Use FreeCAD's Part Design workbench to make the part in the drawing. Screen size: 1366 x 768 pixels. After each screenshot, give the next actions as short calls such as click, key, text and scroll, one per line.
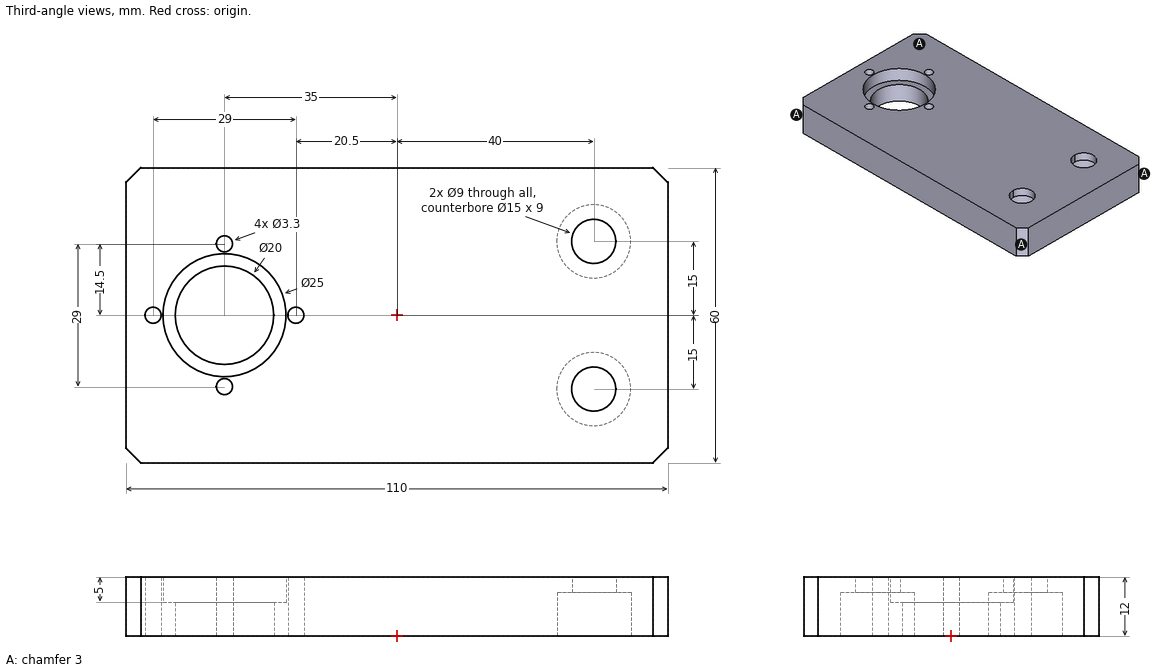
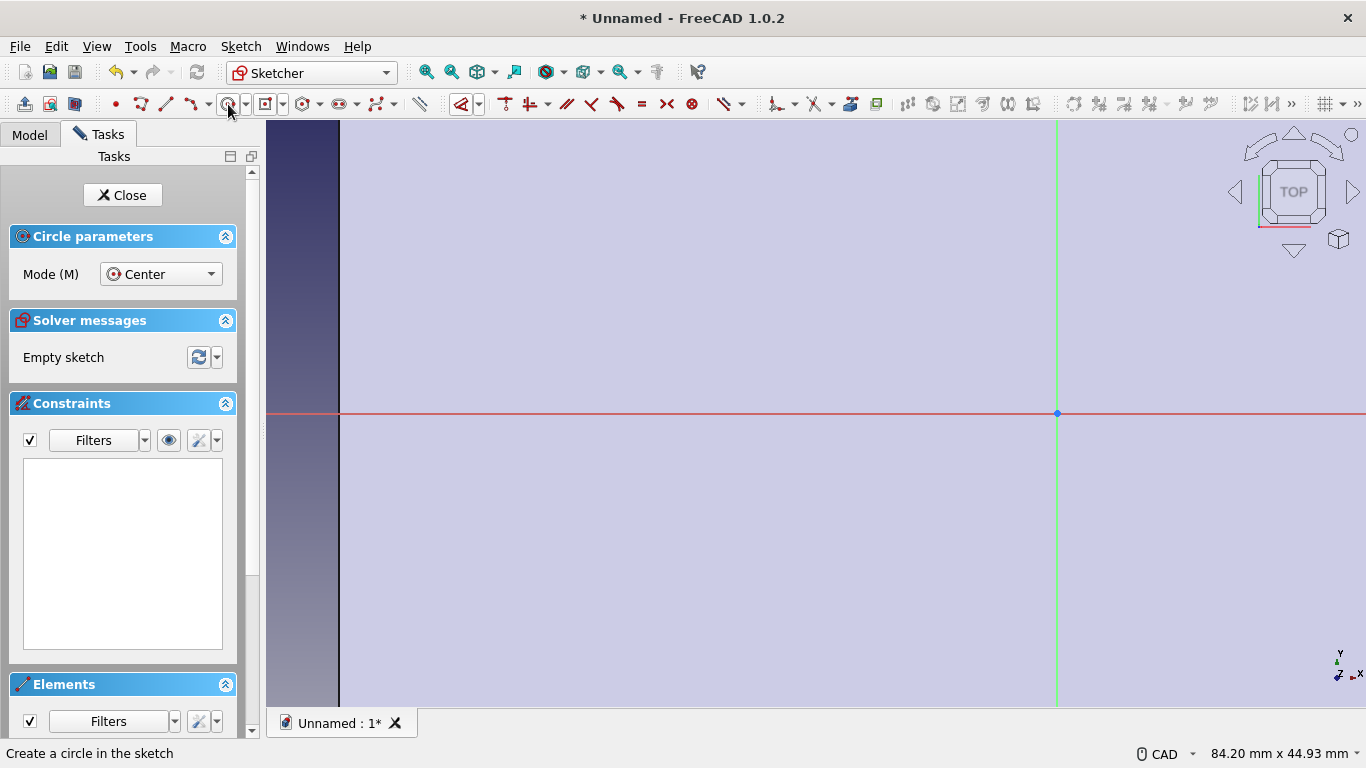
click(600, 414)
click(715, 298)
key(Escape)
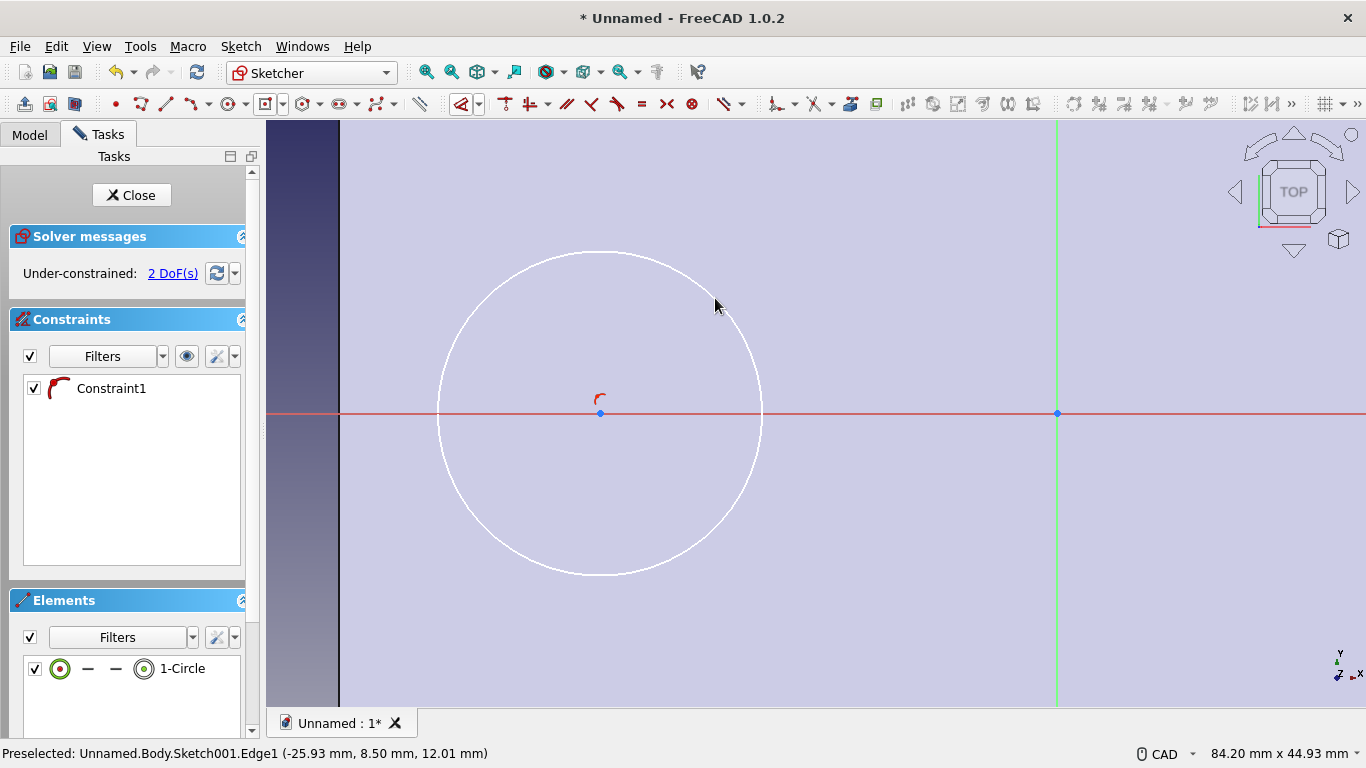
click(460, 104)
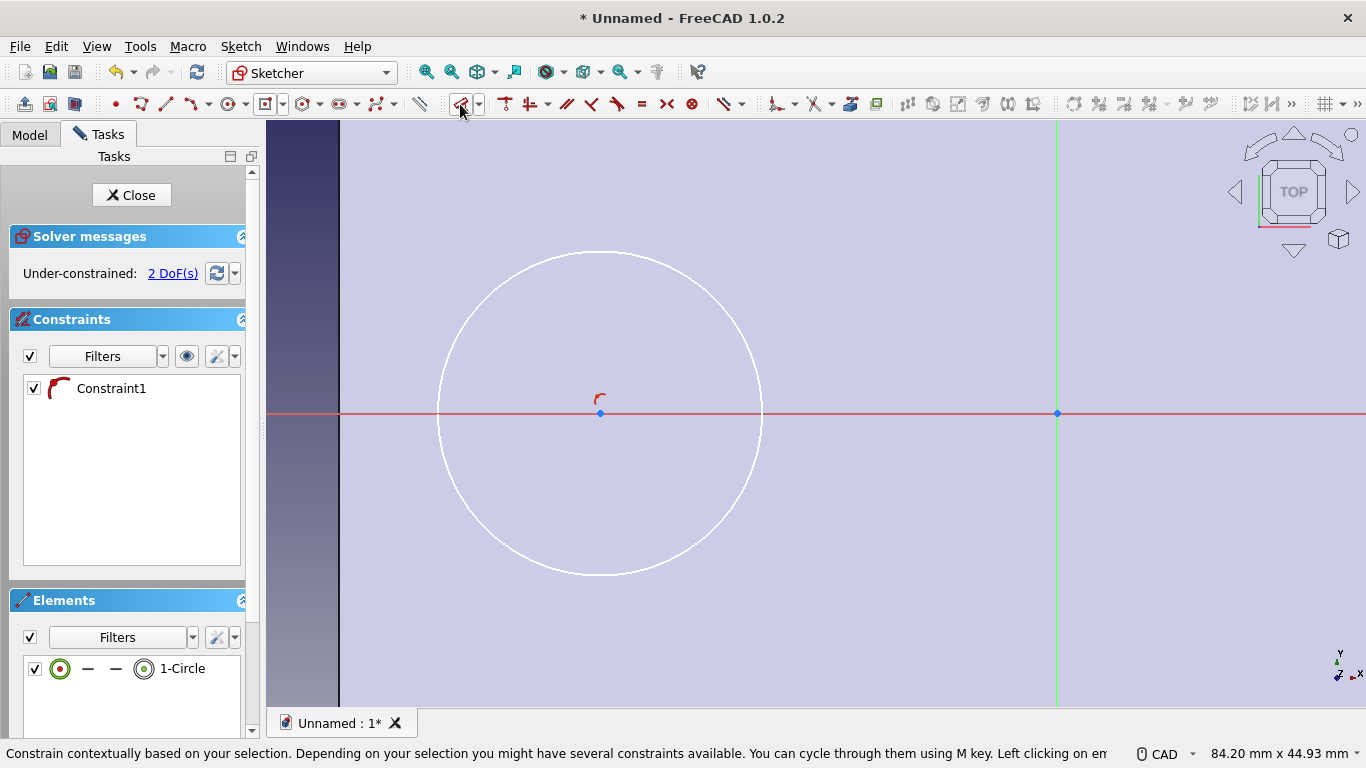
click(714, 298)
click(736, 275)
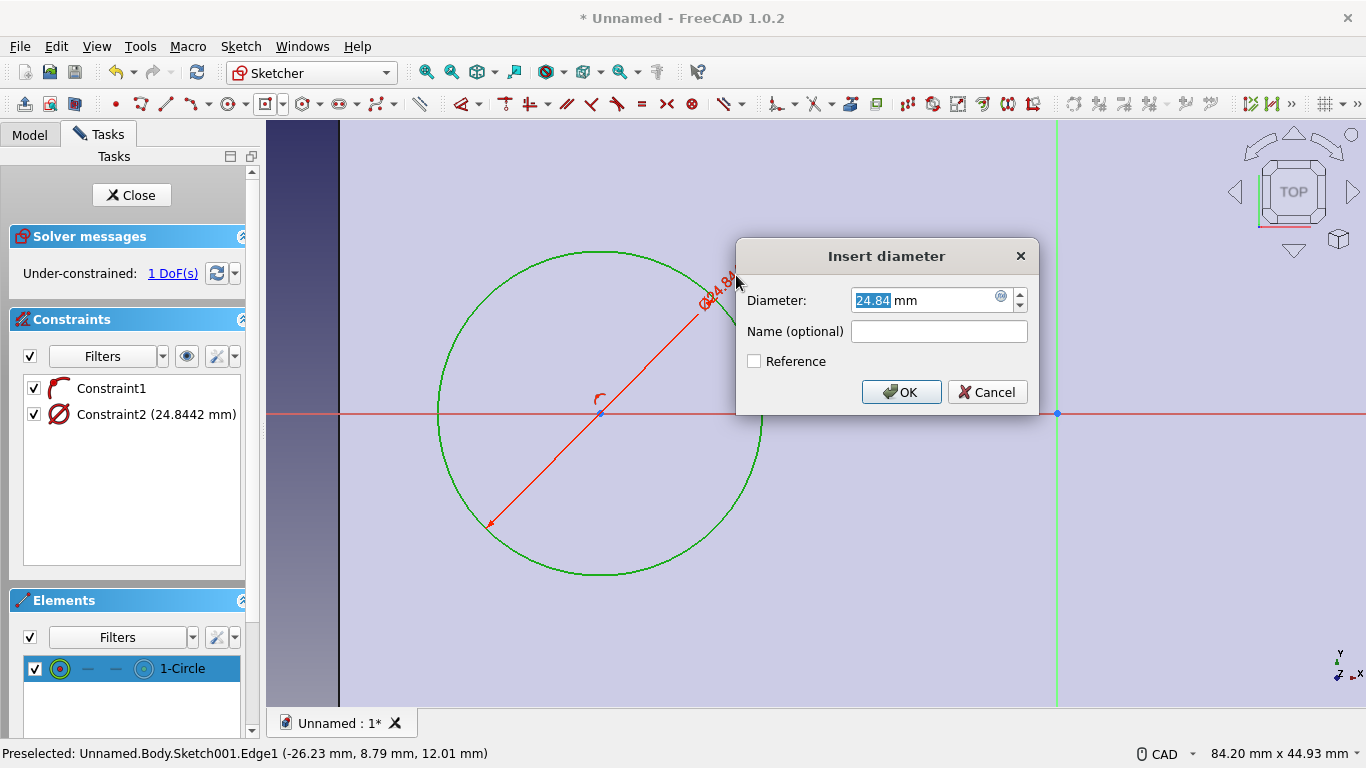
text(25)
key(Return)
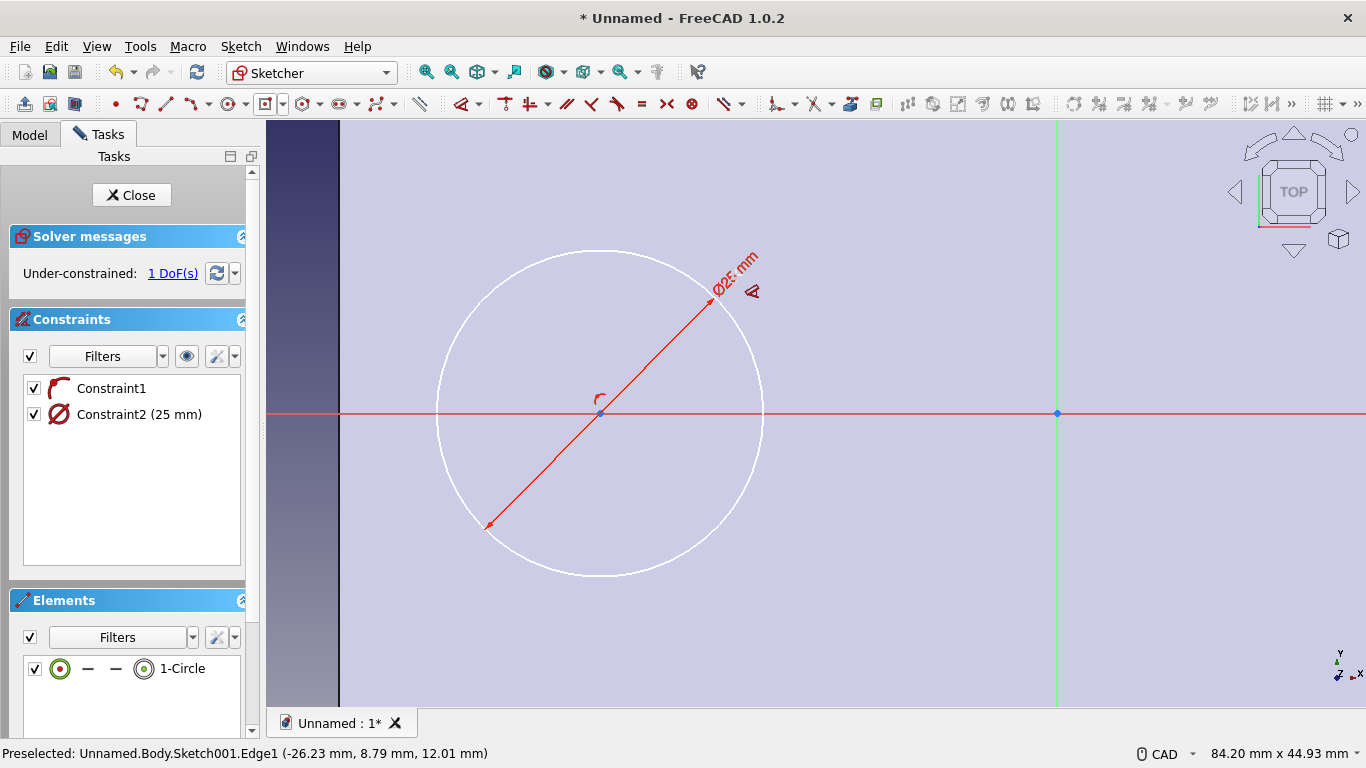
click(600, 414)
click(829, 448)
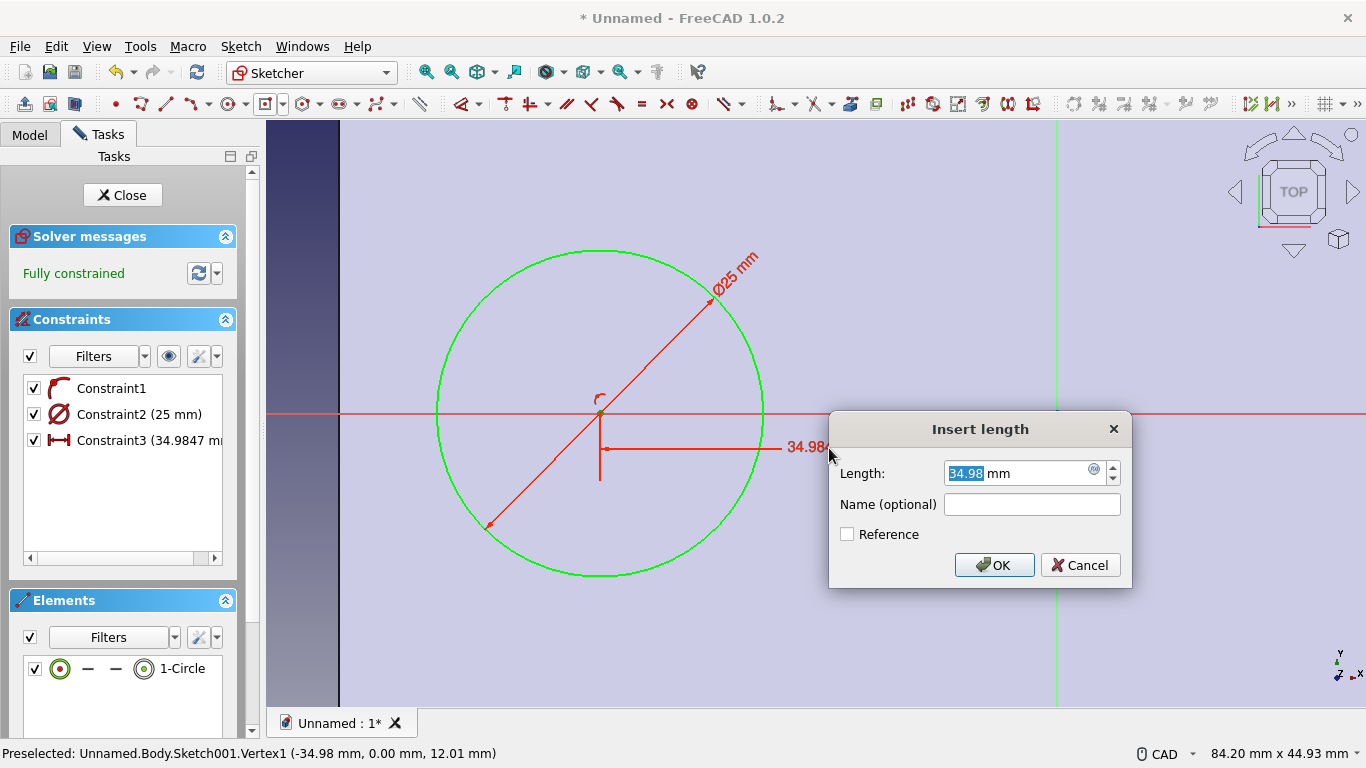
text(35)
key(Return)
key(Escape)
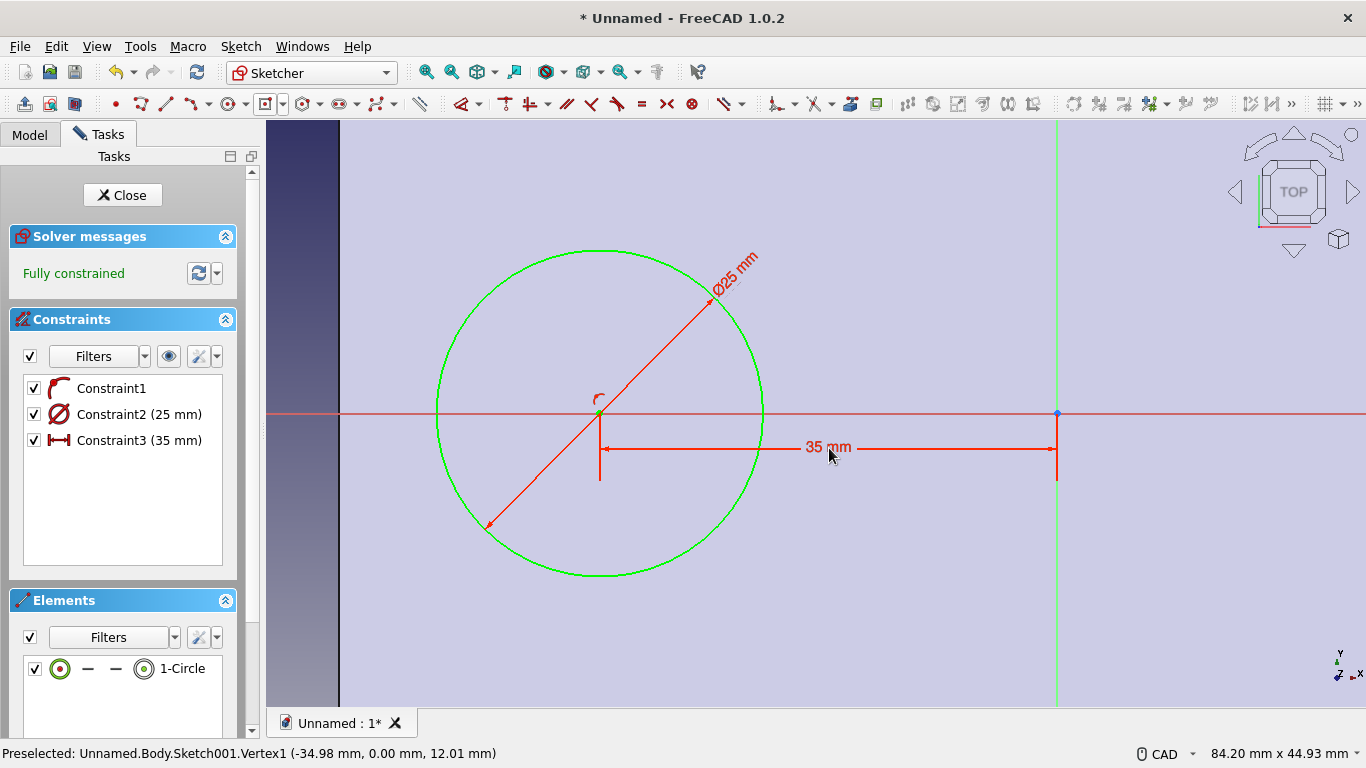
click(123, 195)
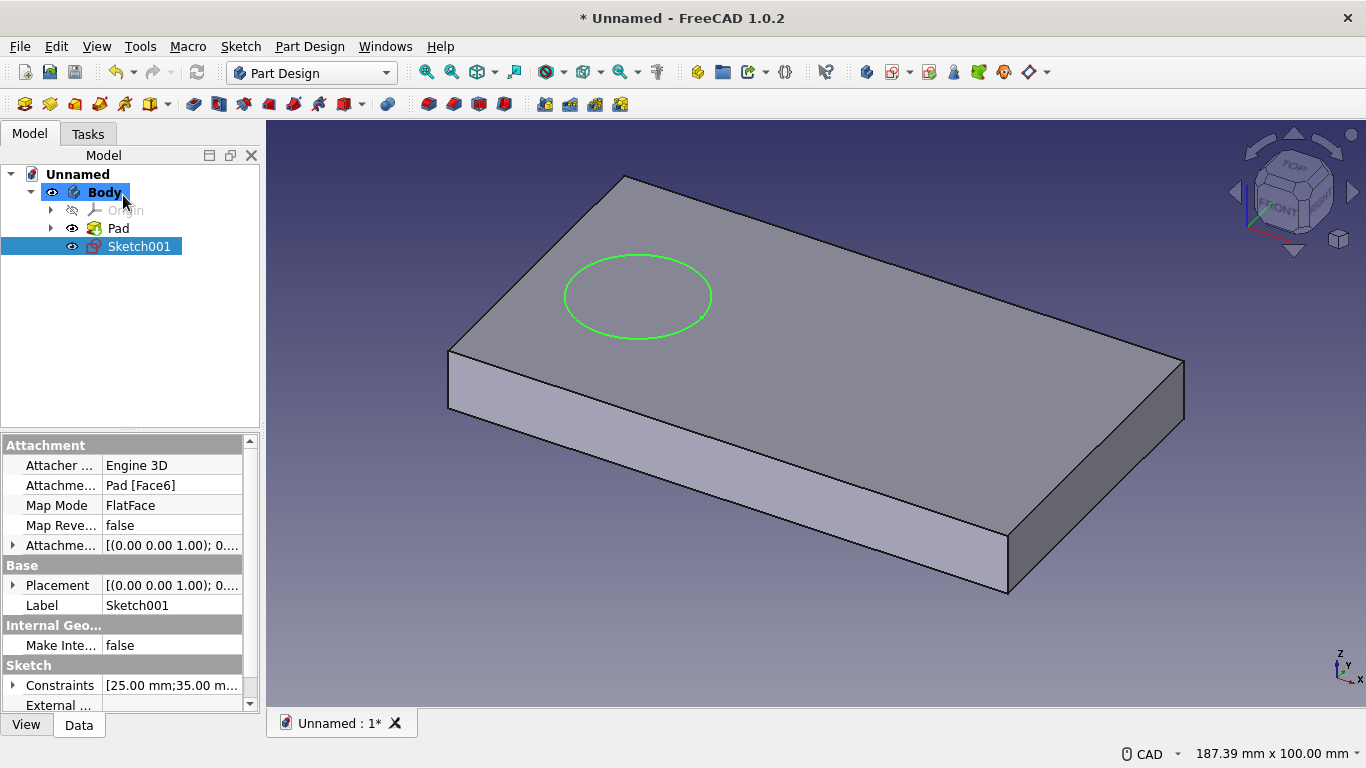
click(194, 104)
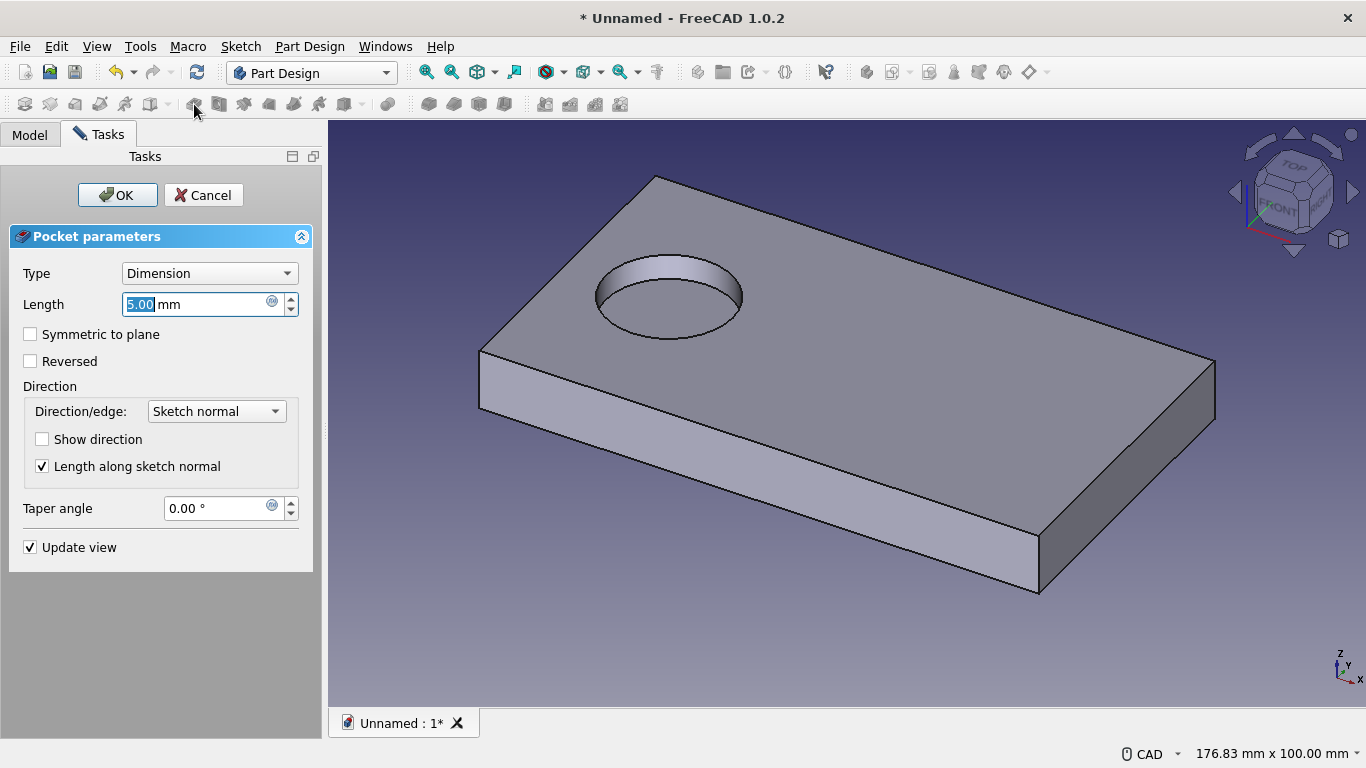
text(5)
key(Tab)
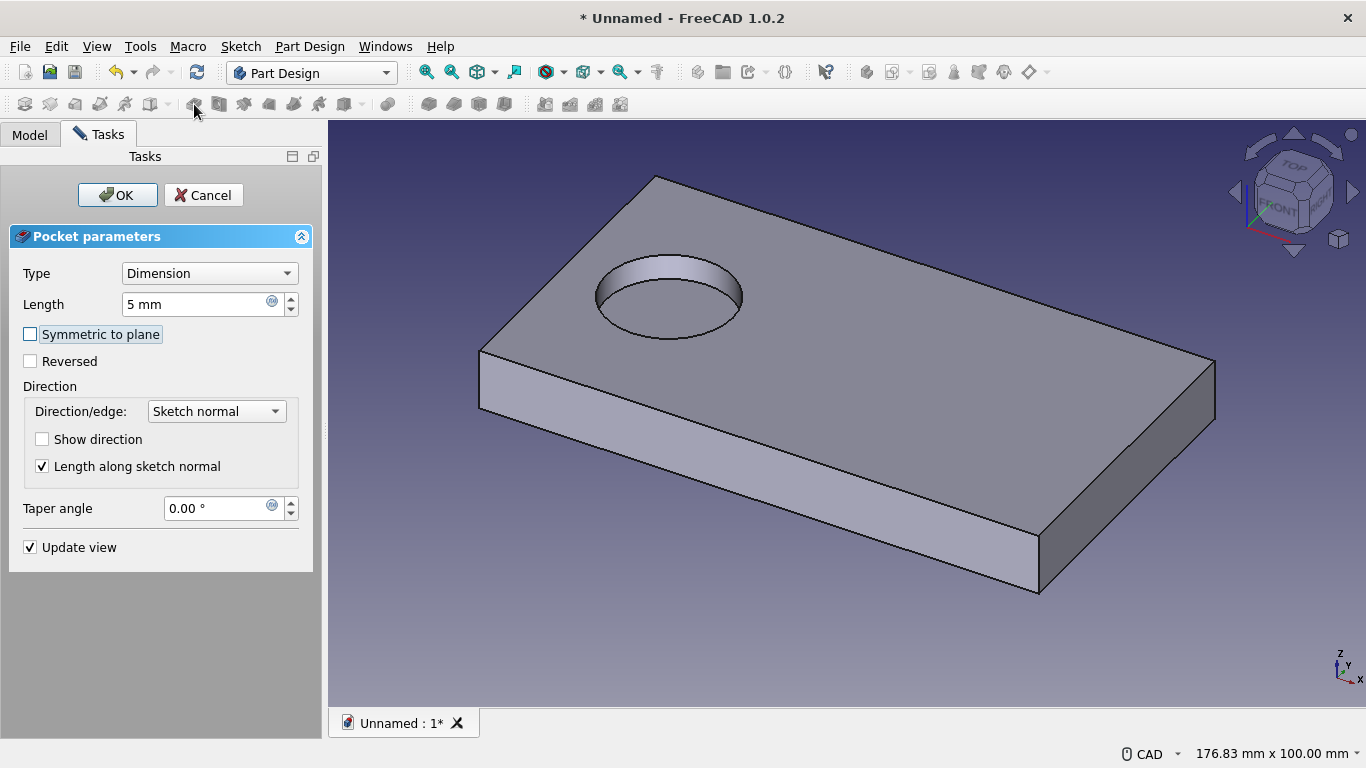
click(118, 195)